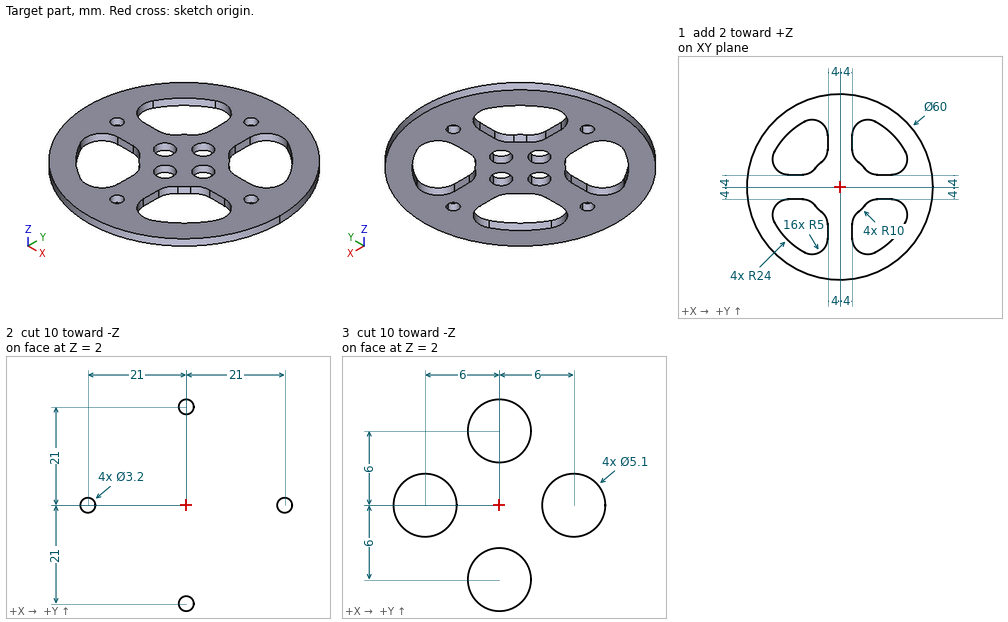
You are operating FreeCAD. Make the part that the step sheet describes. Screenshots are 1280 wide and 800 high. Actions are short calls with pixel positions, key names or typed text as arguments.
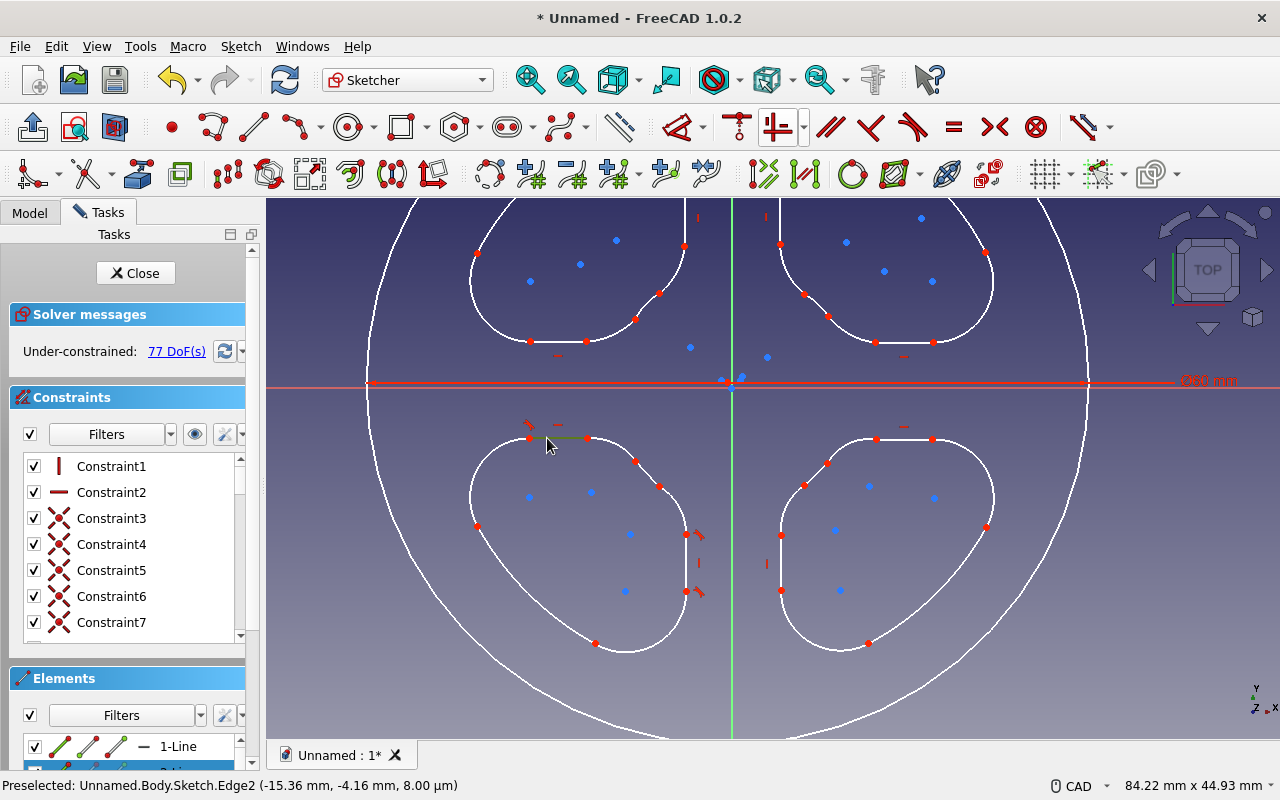
click(624, 449)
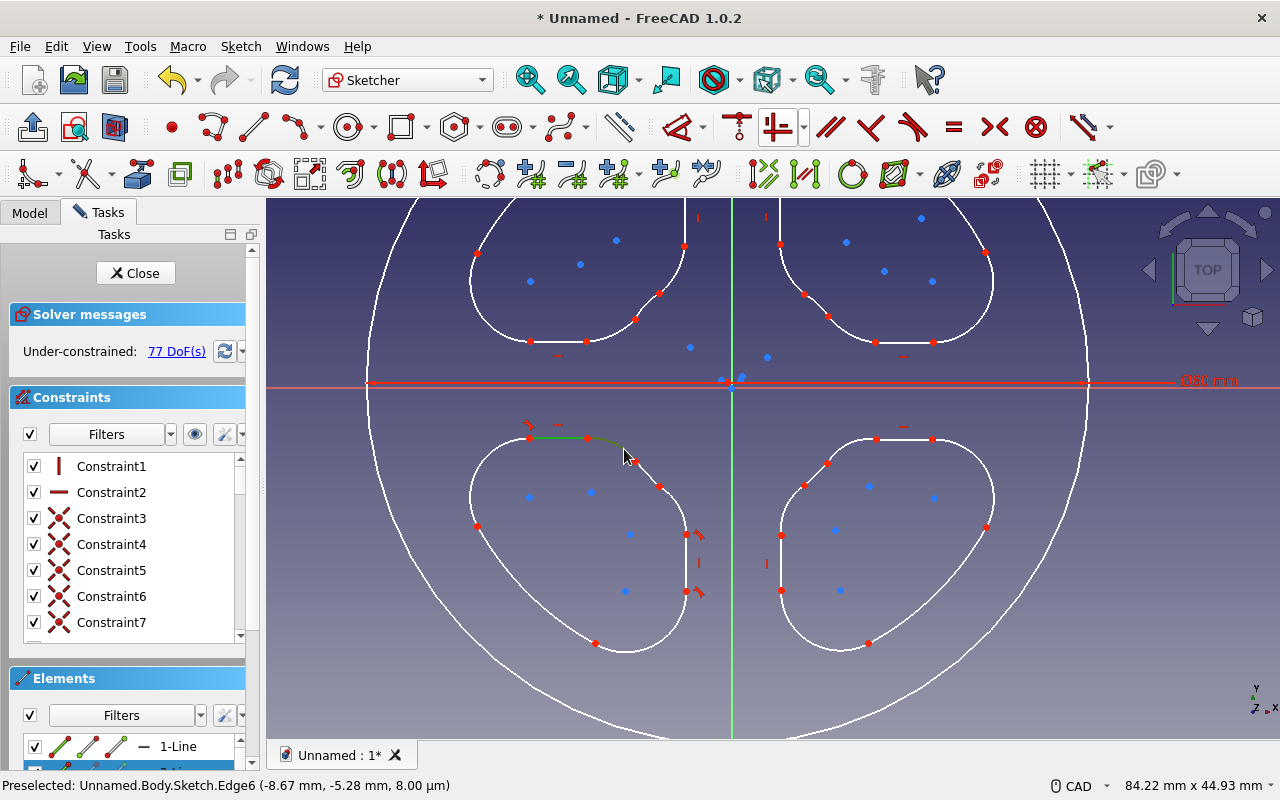
click(913, 128)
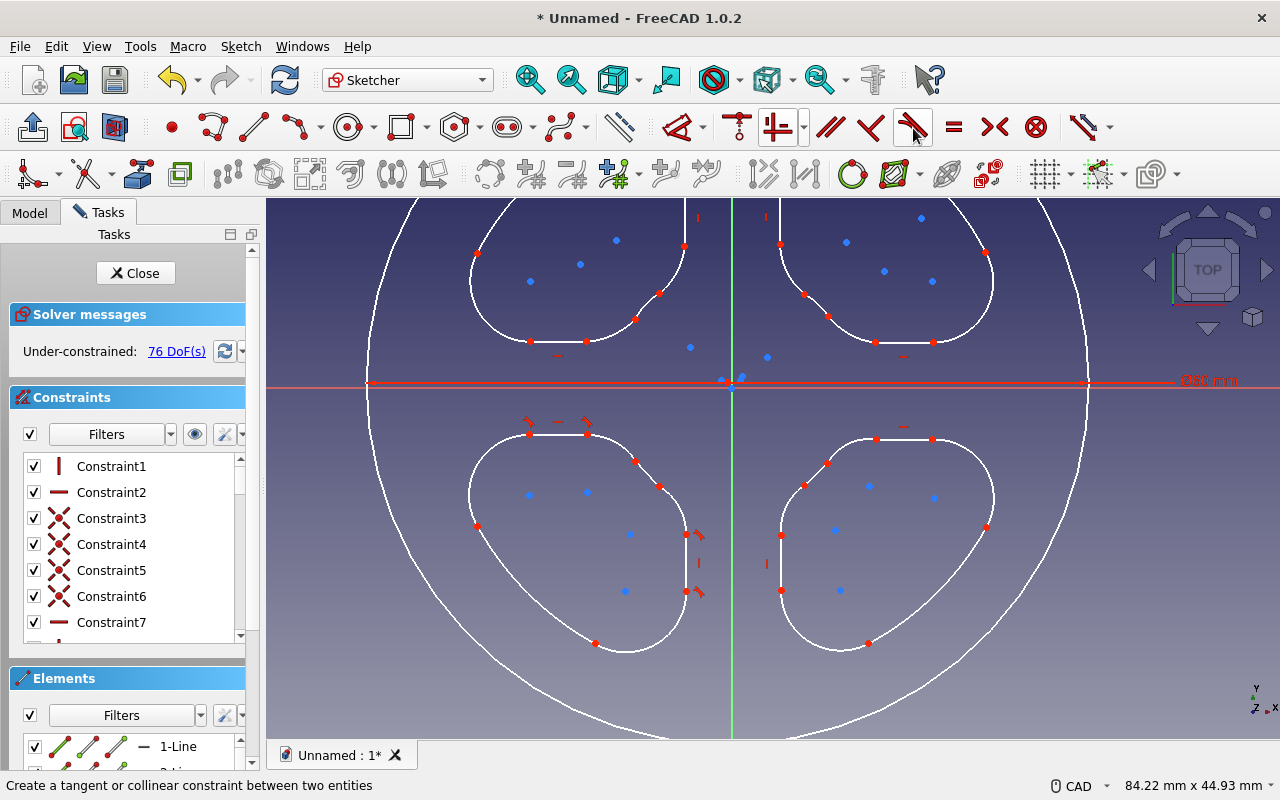
click(632, 652)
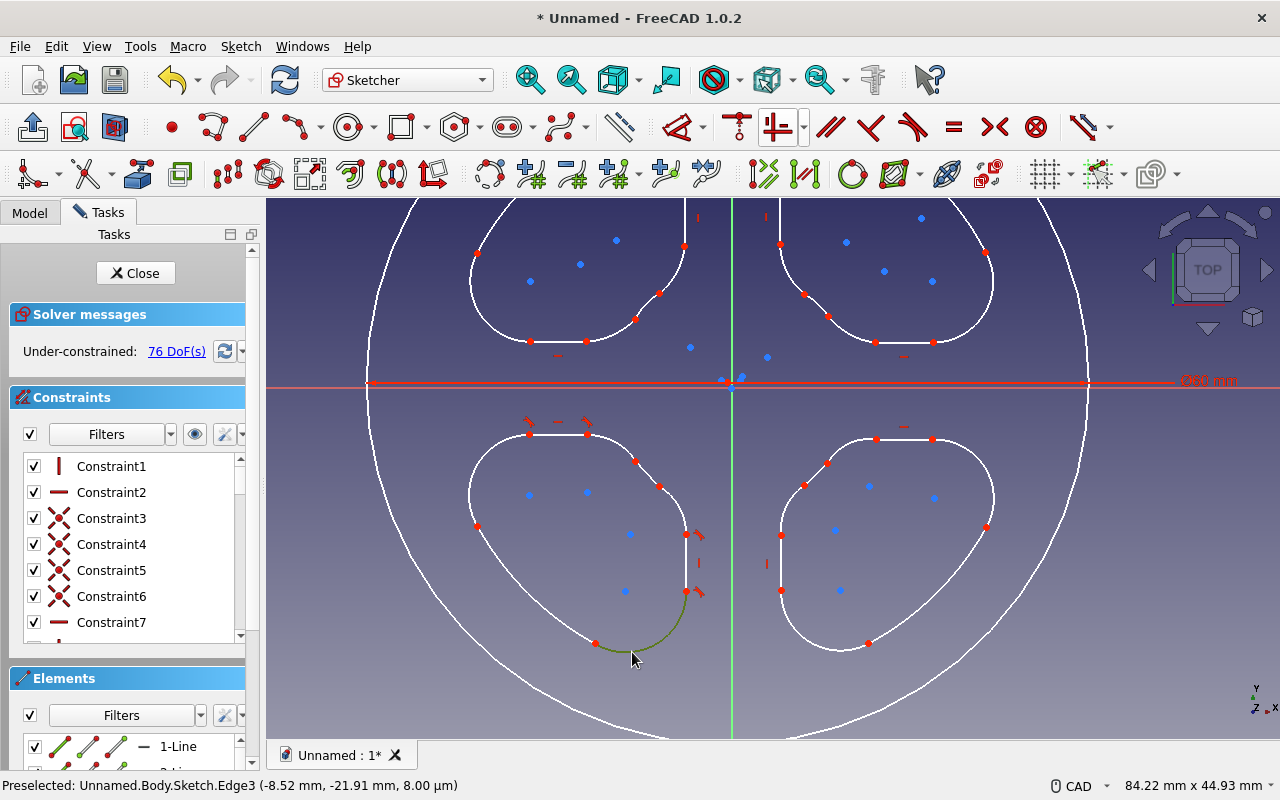
click(506, 568)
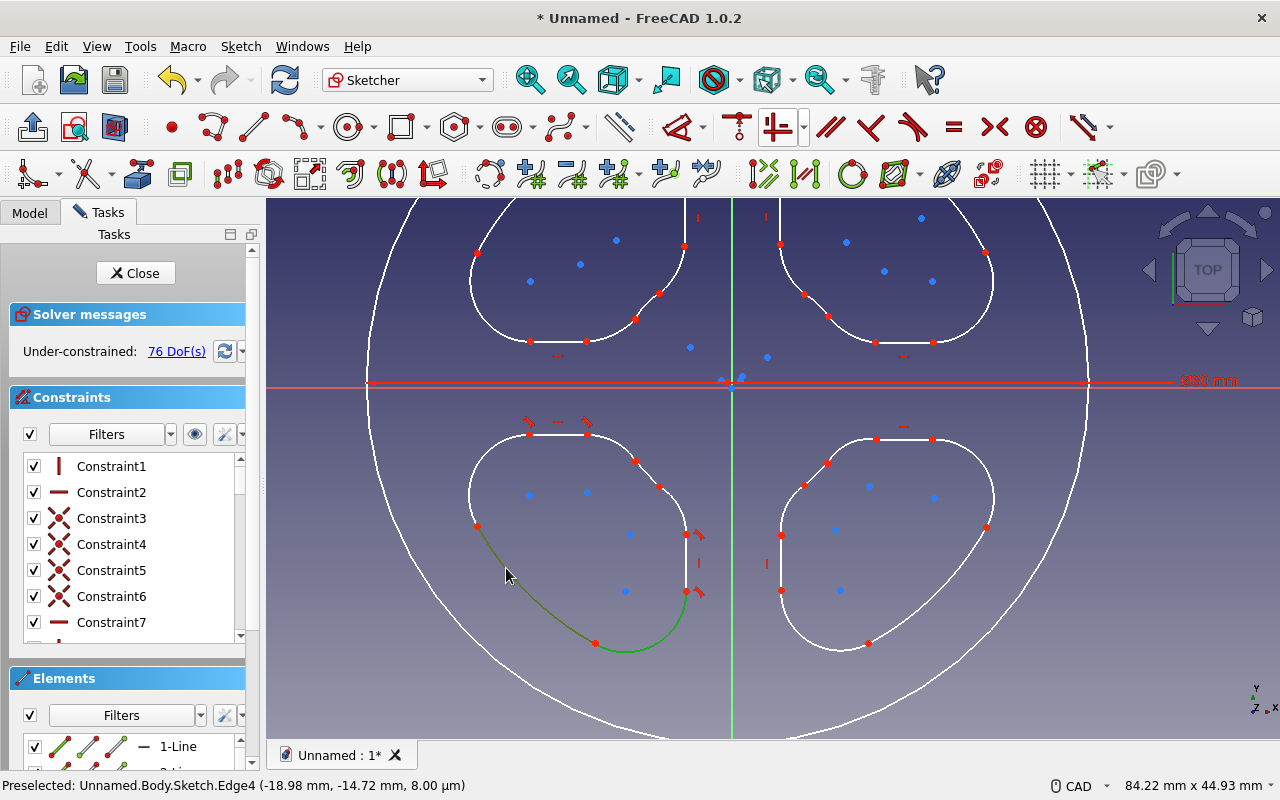
click(913, 128)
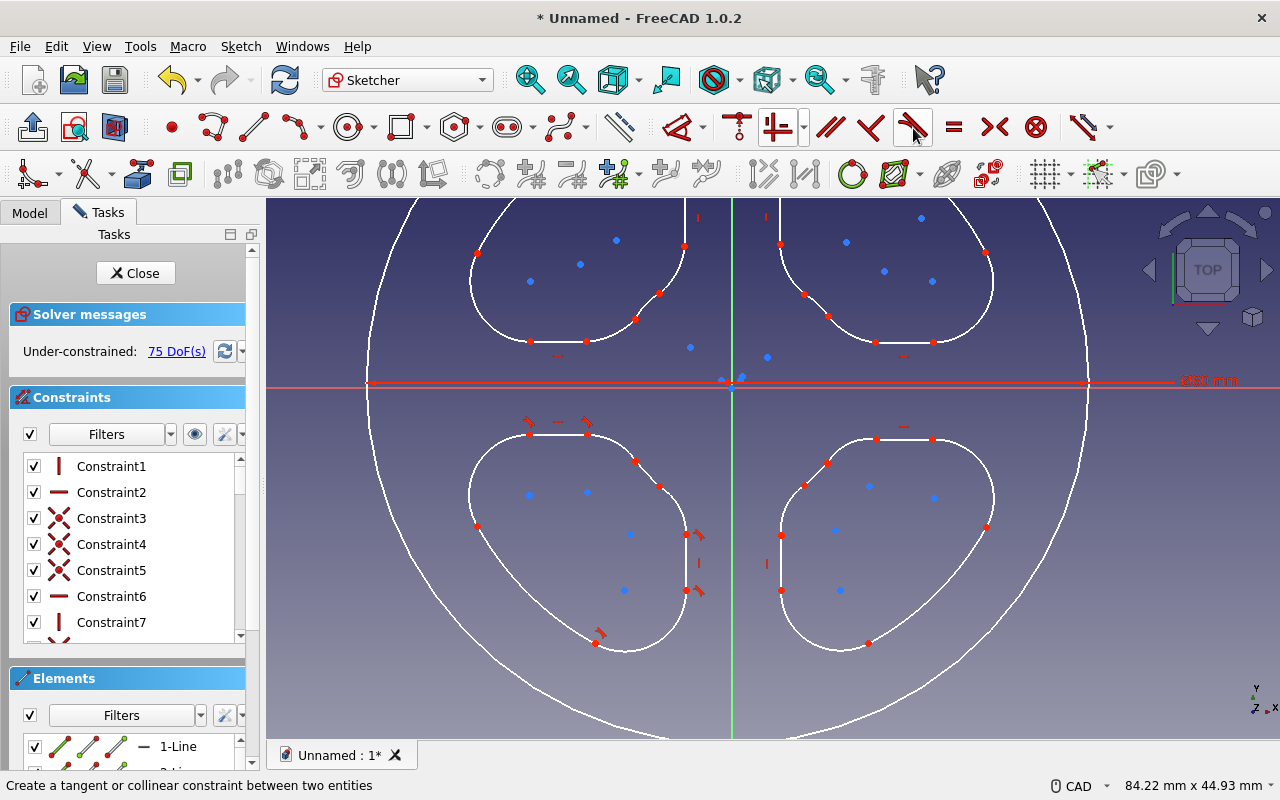
click(506, 568)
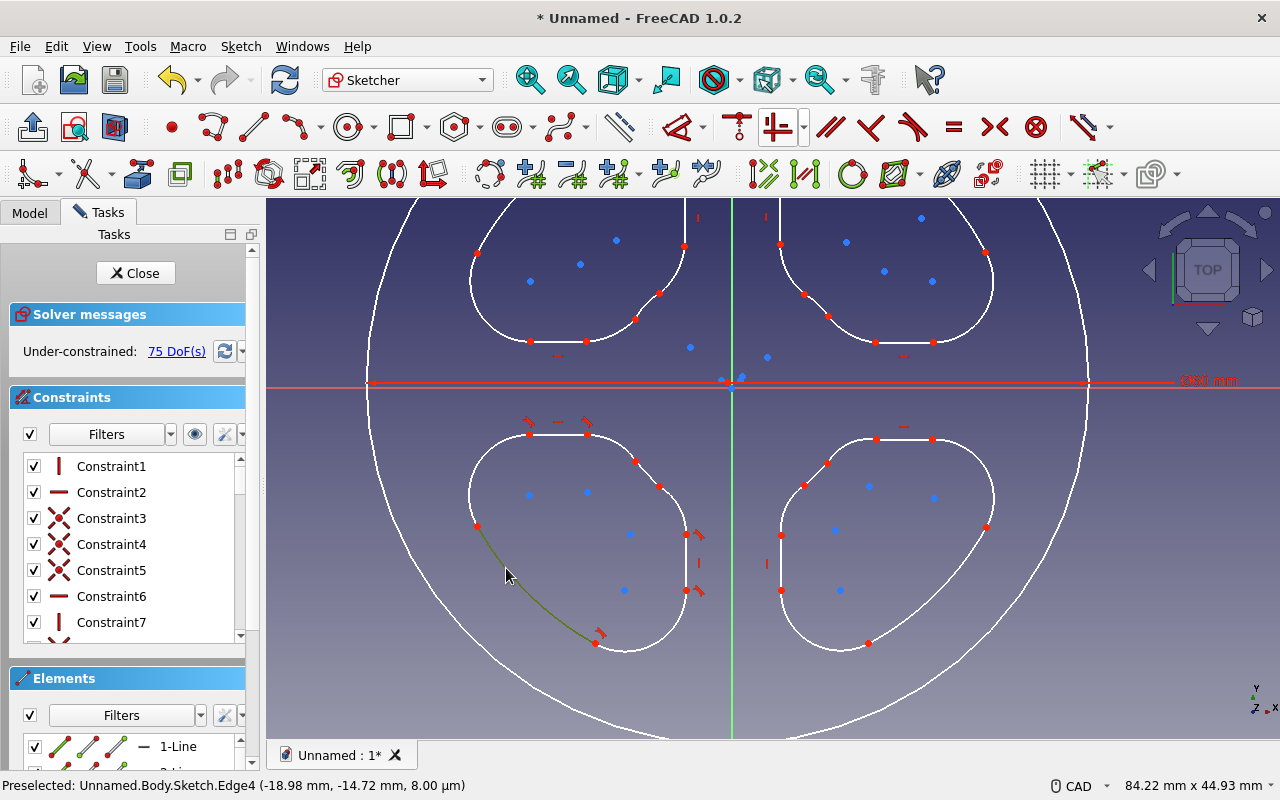
click(494, 447)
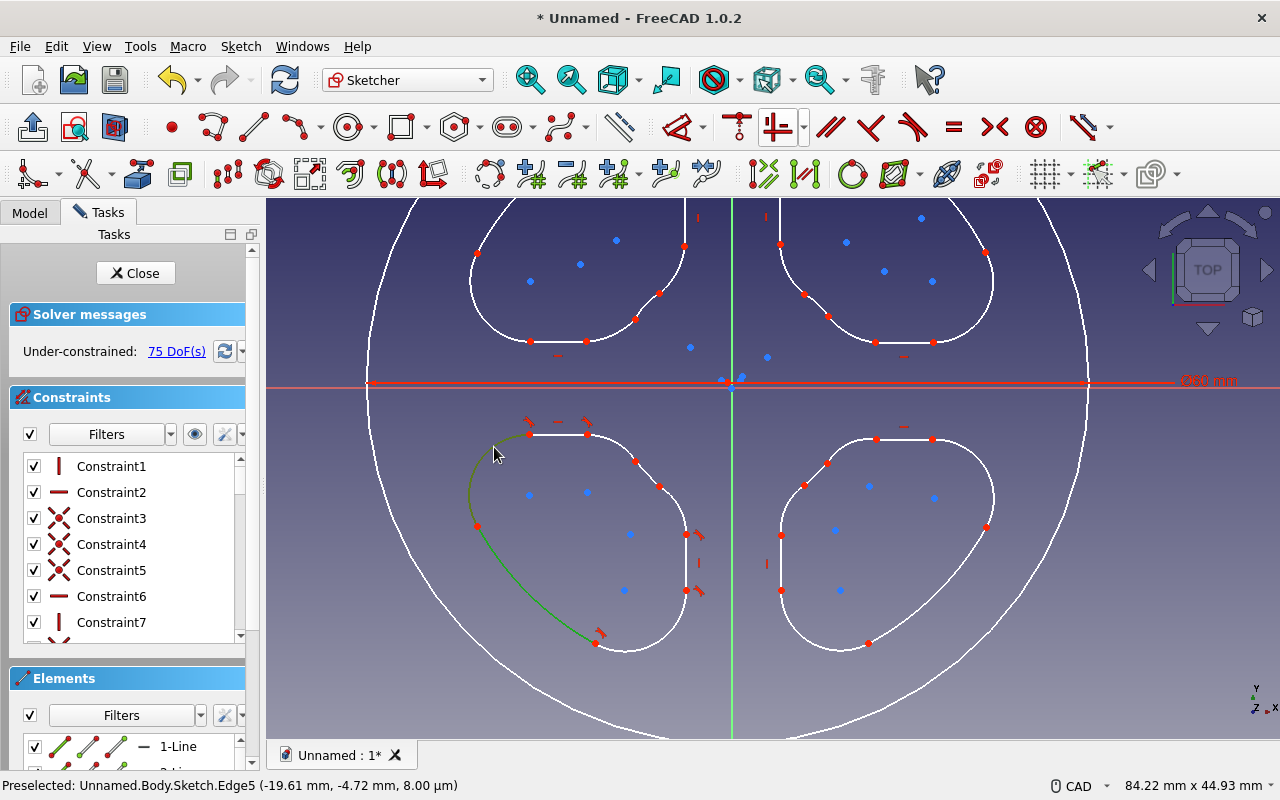
click(913, 128)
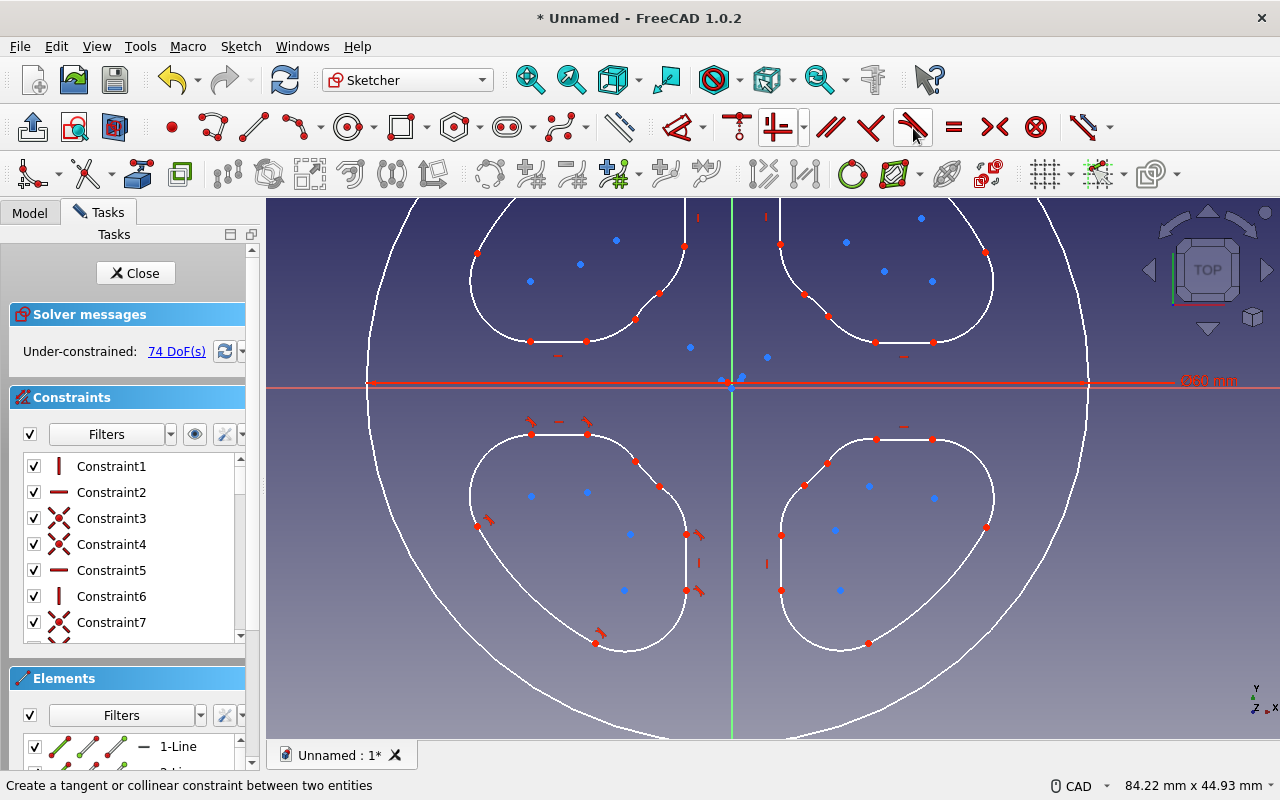
click(624, 448)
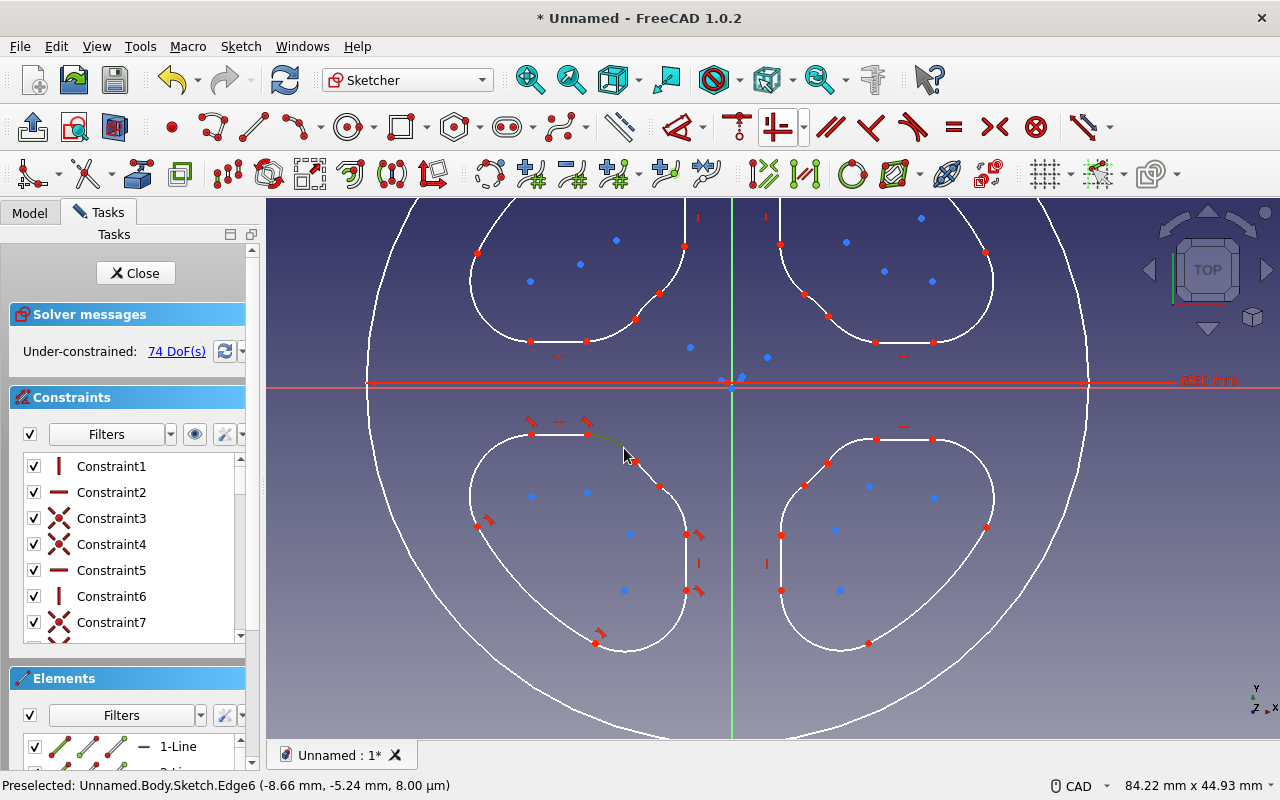
scroll(643, 469, up, 2)